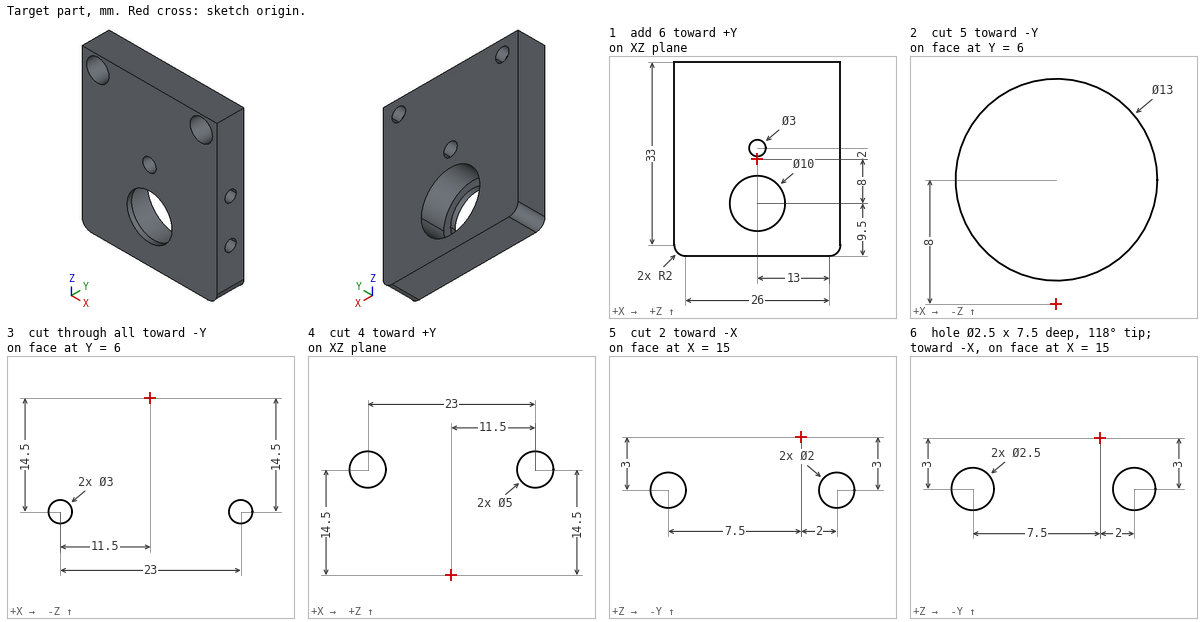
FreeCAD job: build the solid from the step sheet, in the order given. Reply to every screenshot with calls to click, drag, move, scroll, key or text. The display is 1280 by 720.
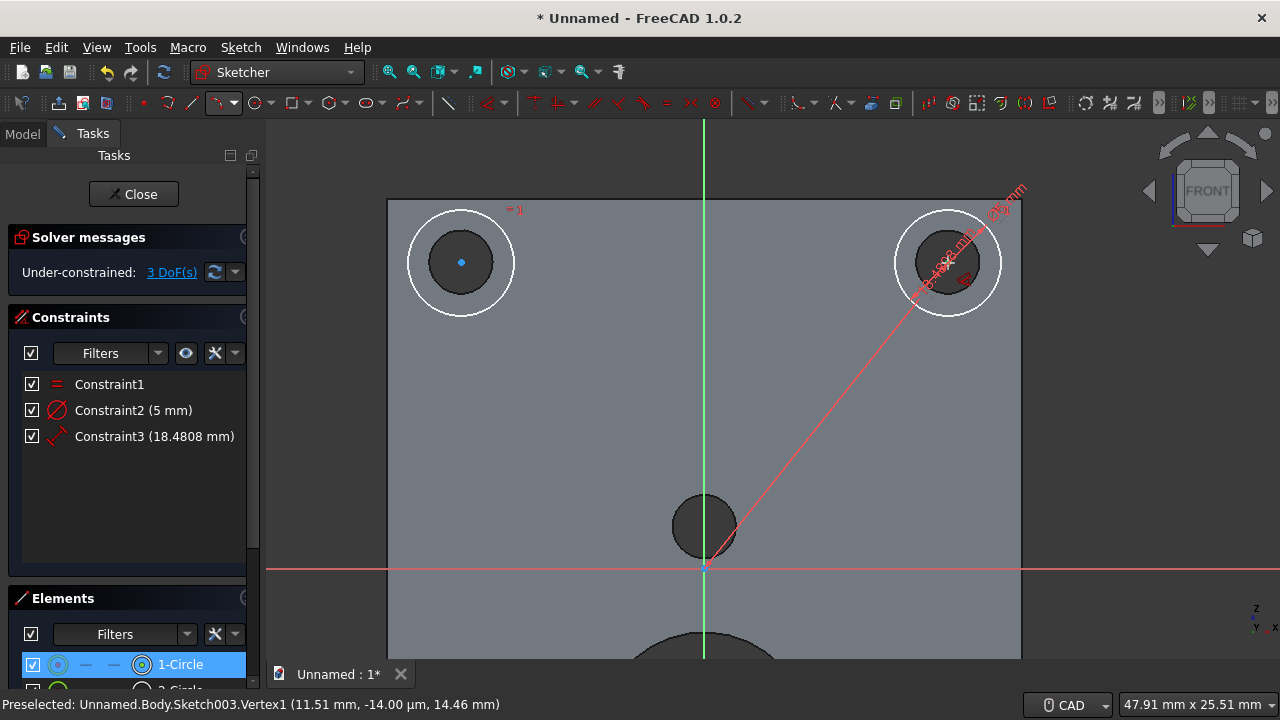
click(461, 263)
click(592, 229)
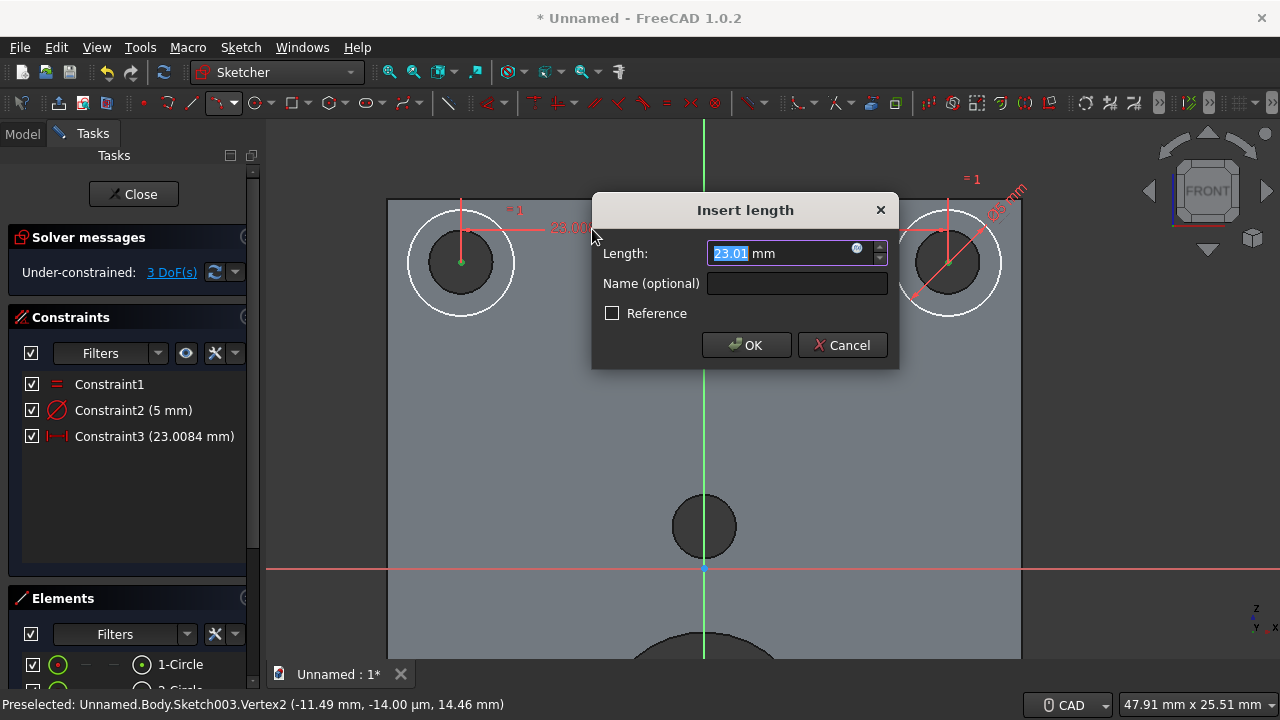
text(23)
key(Return)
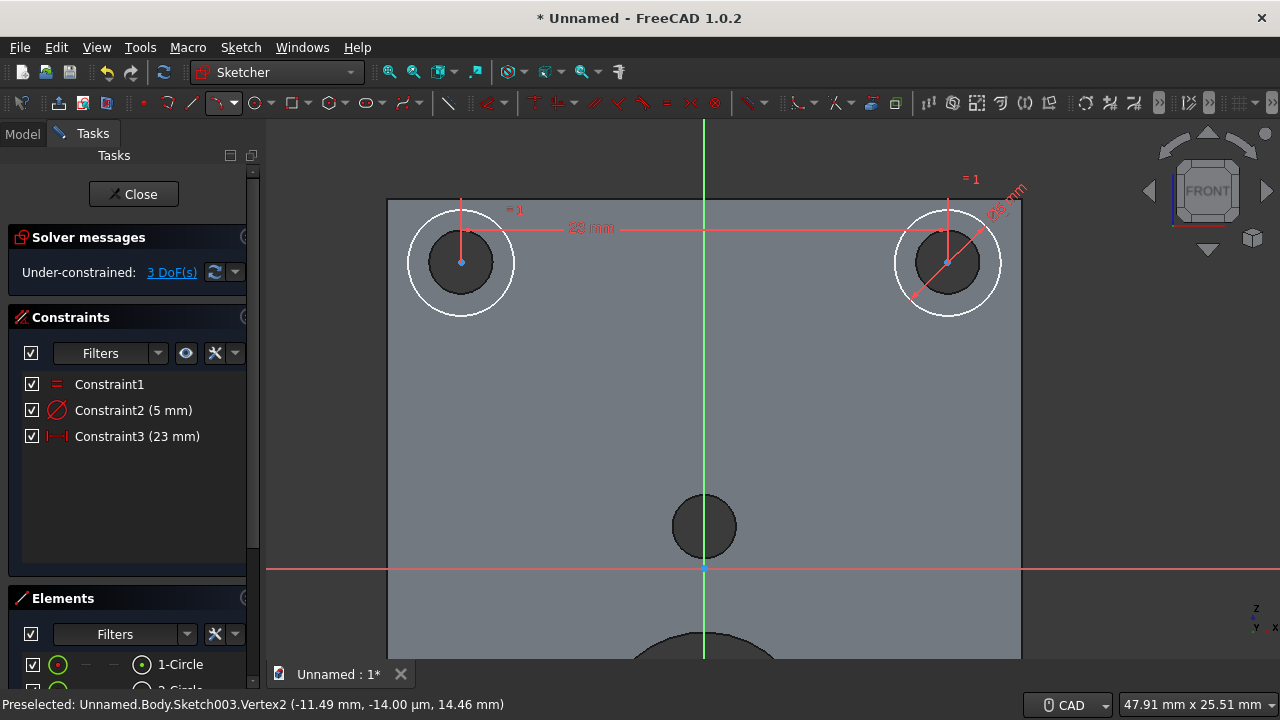
click(948, 263)
click(826, 603)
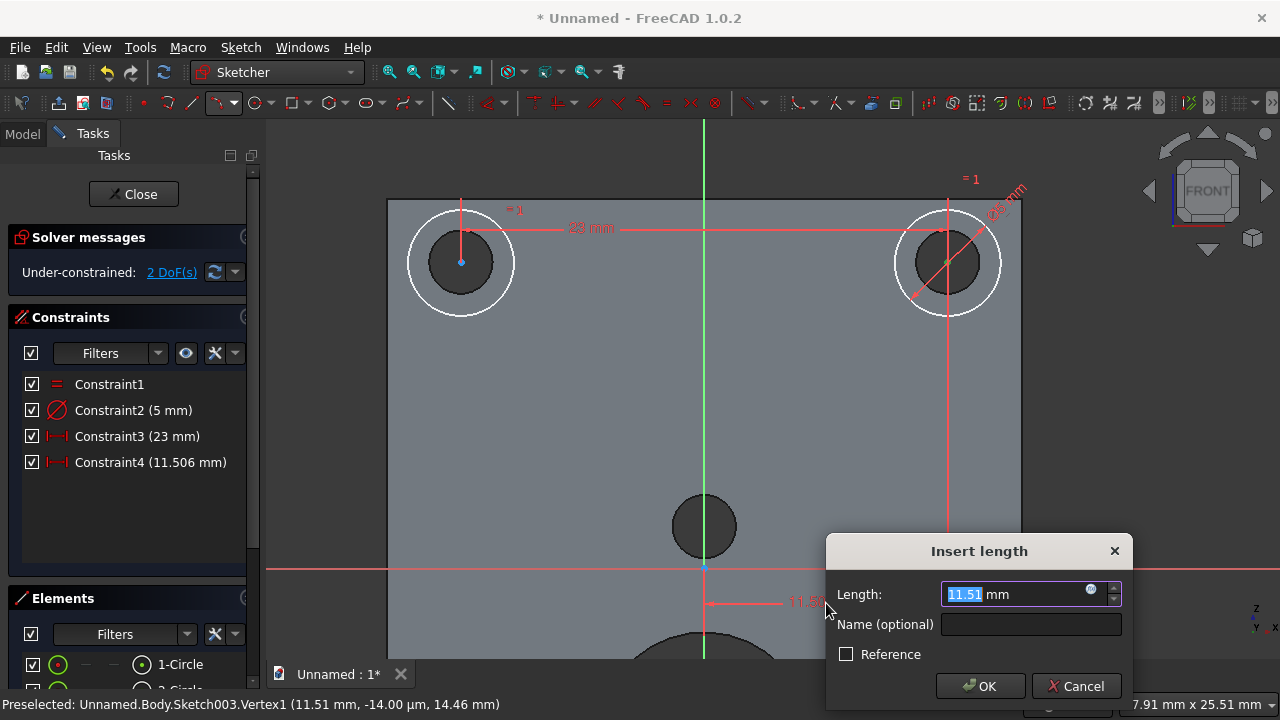
text(11.5)
key(Return)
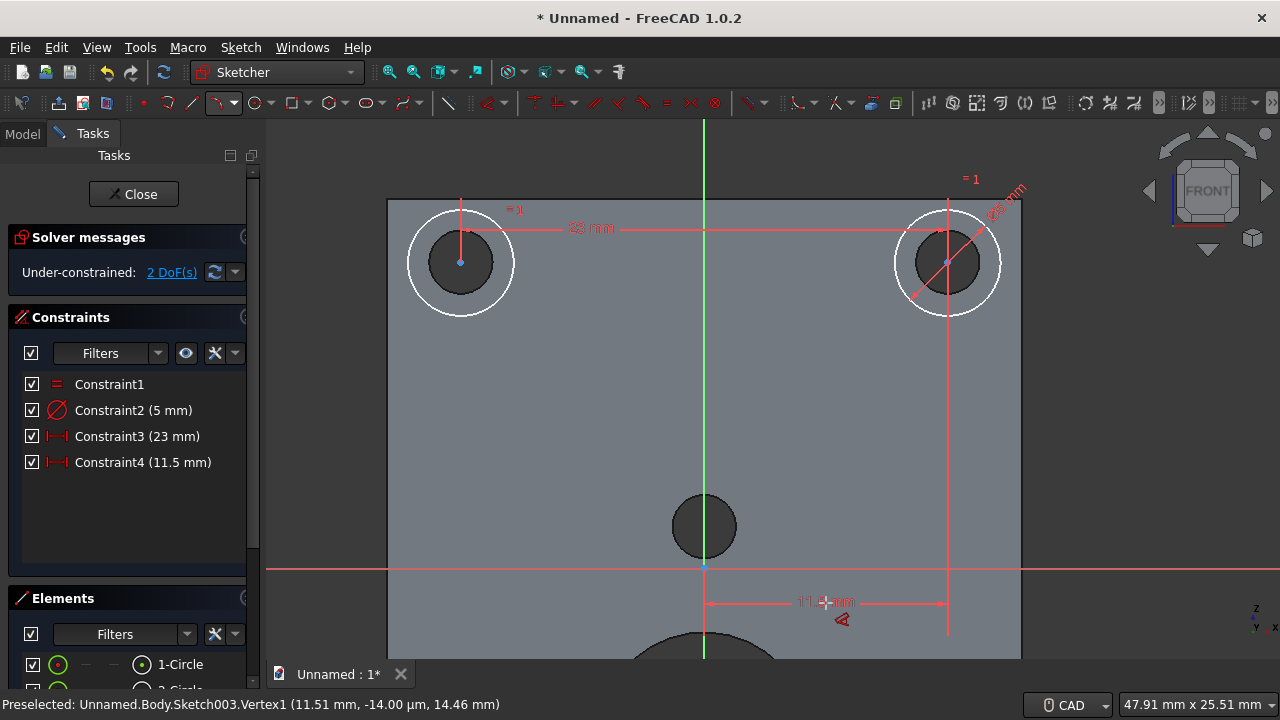
click(948, 263)
click(982, 416)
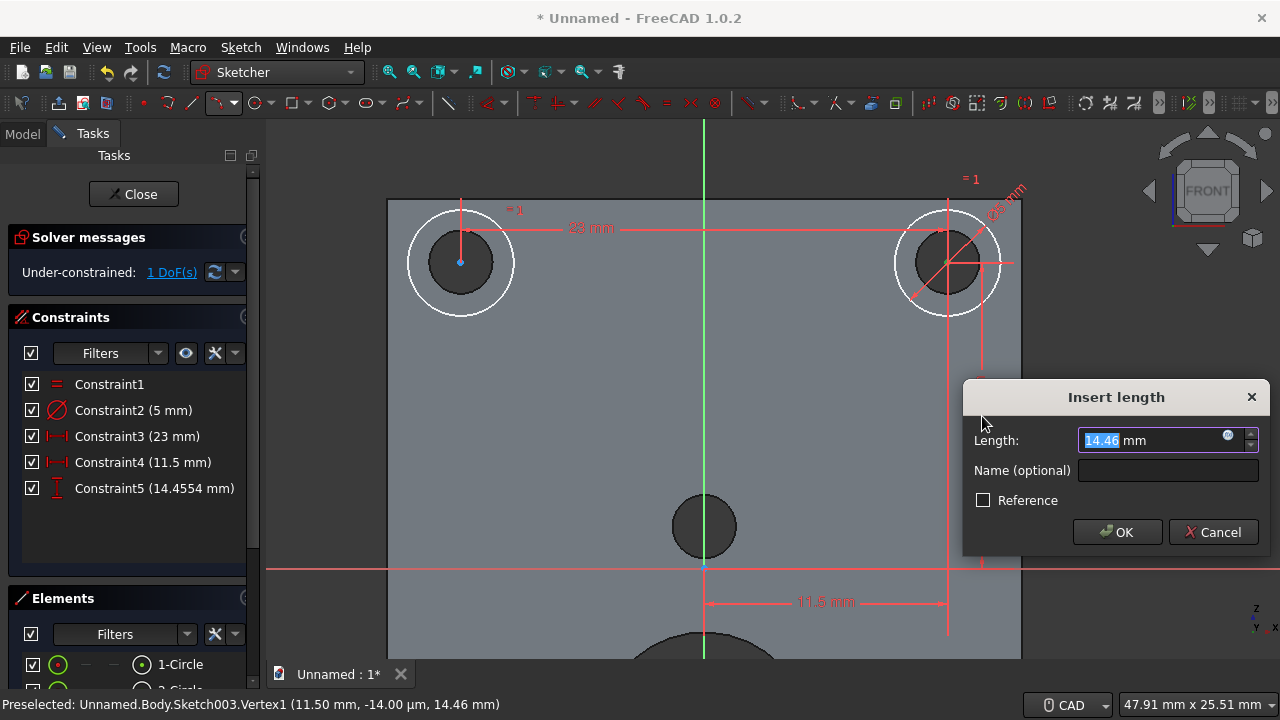
text(14.5)
key(Return)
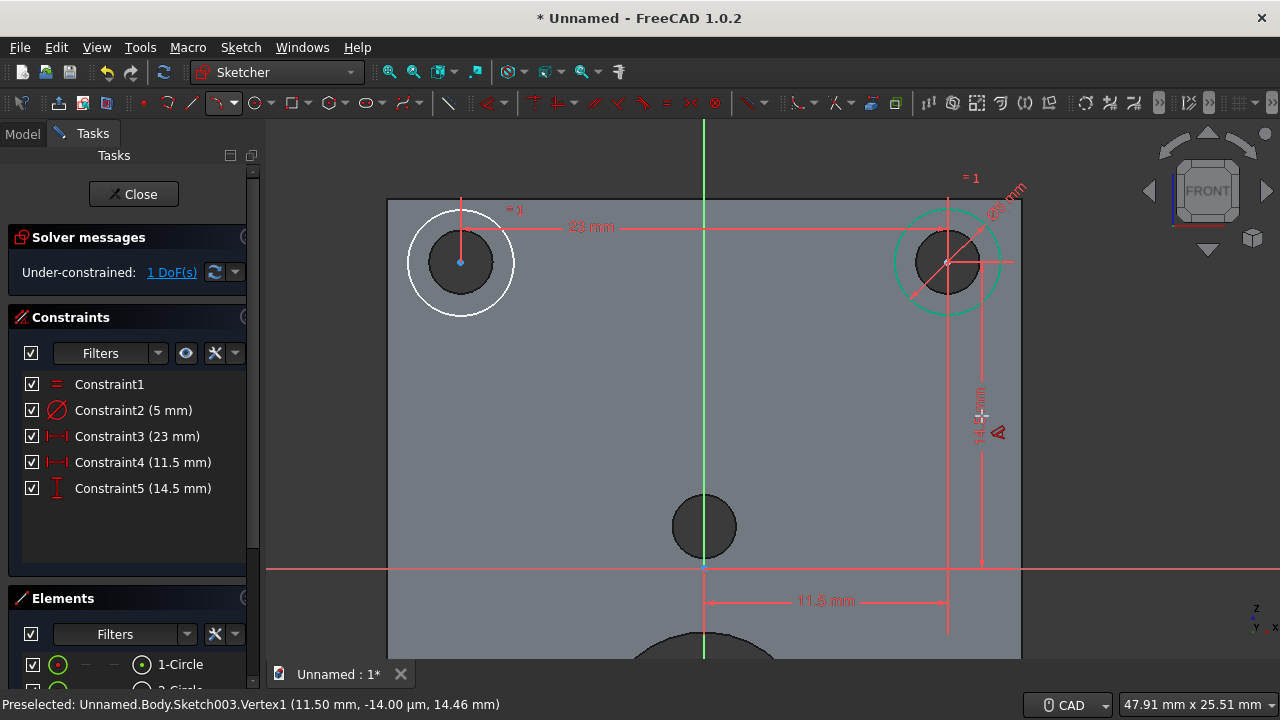
click(461, 263)
click(427, 416)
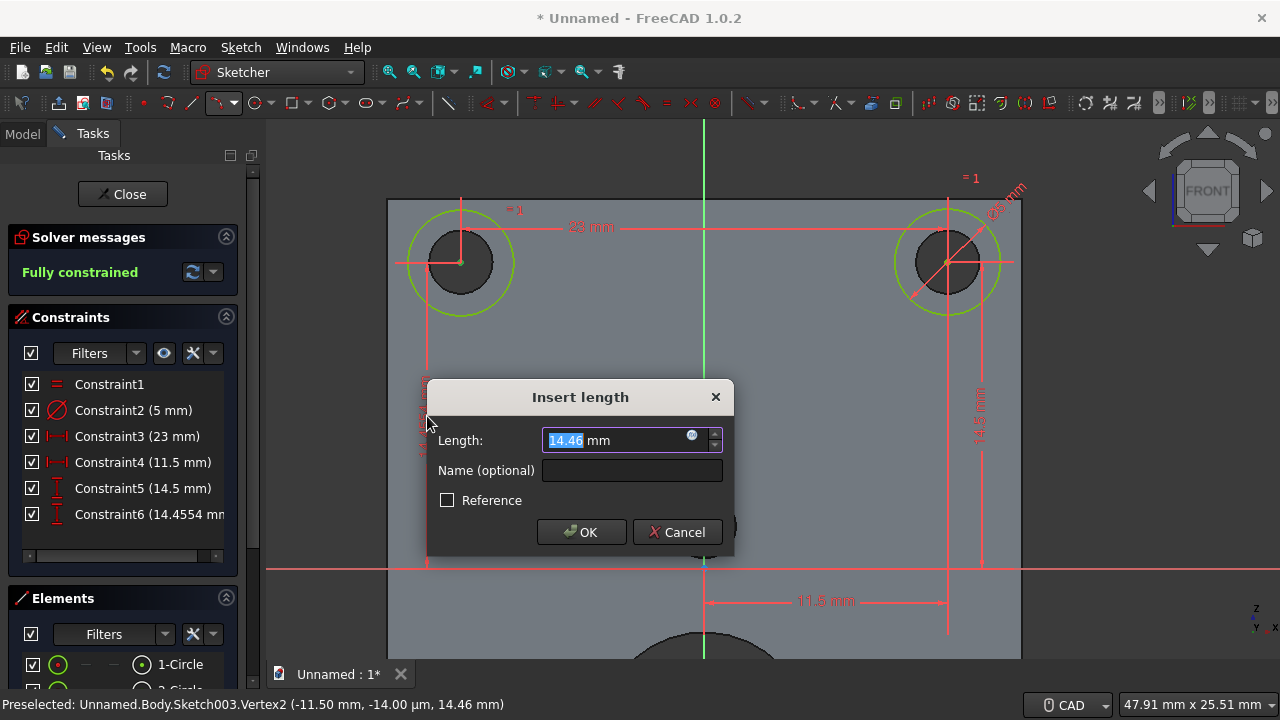
text(14.5)
key(Return)
key(Escape)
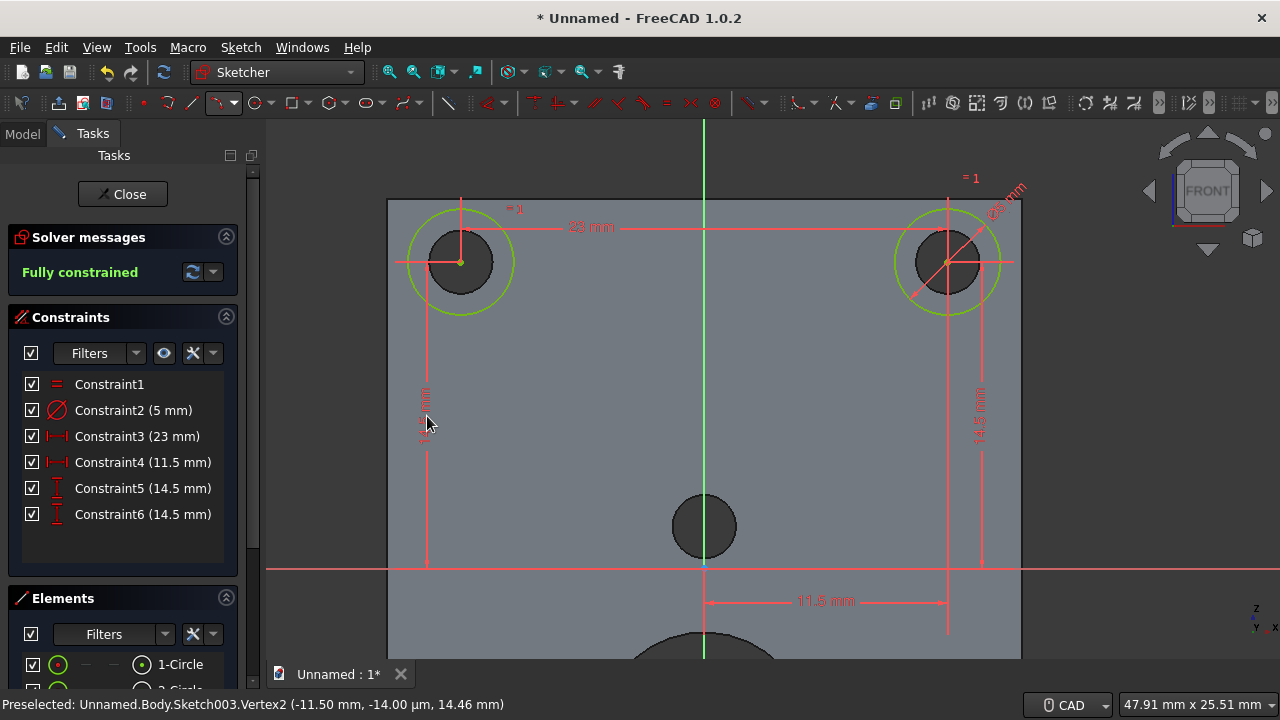
click(123, 194)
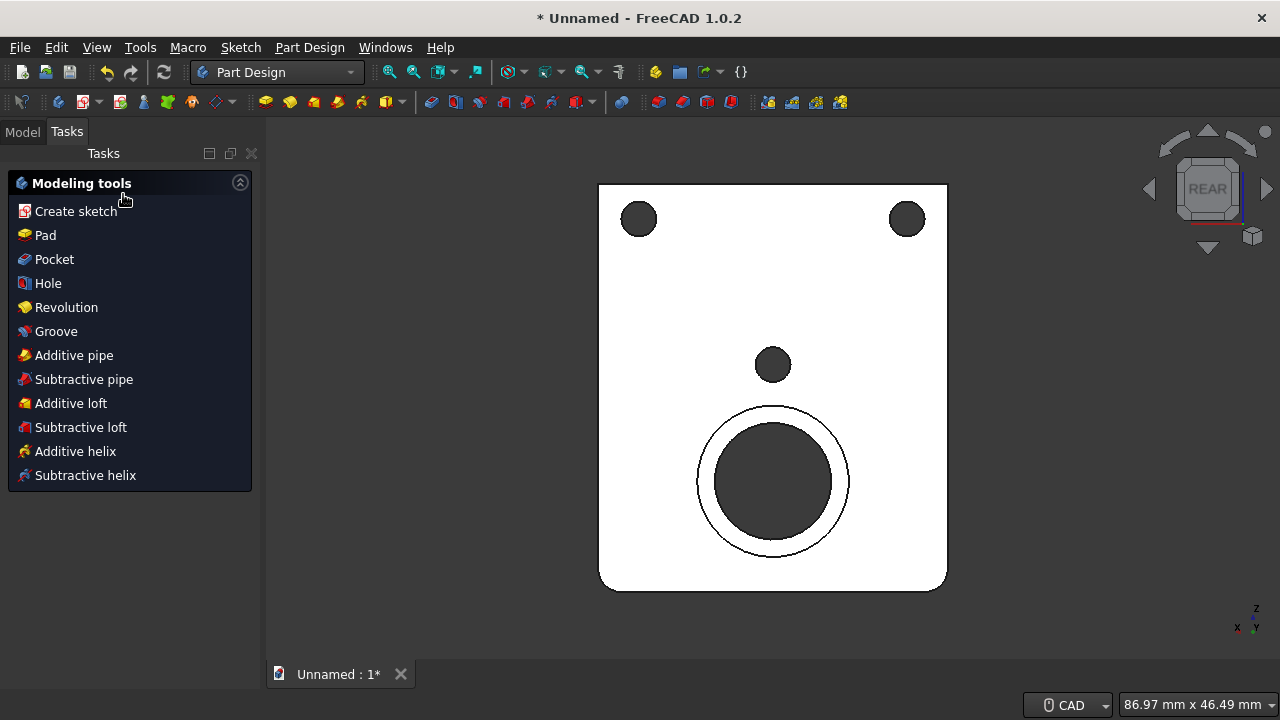
click(432, 102)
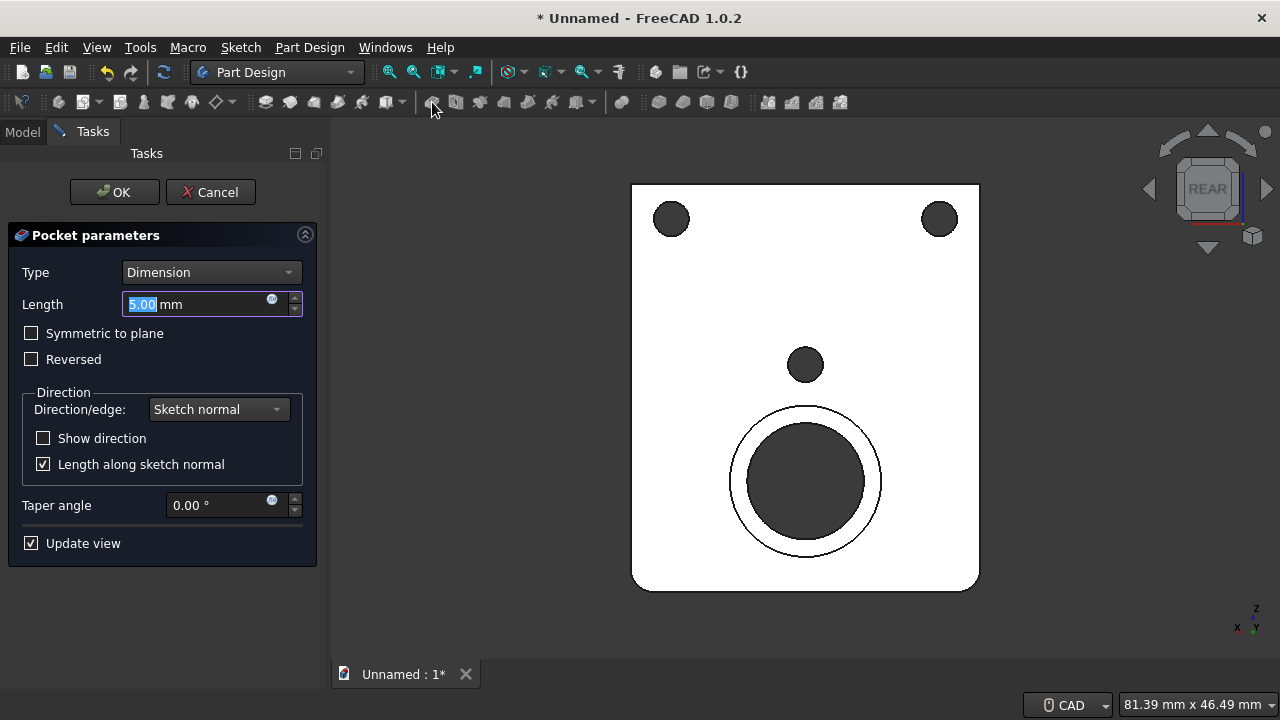
text(4)
key(Tab)